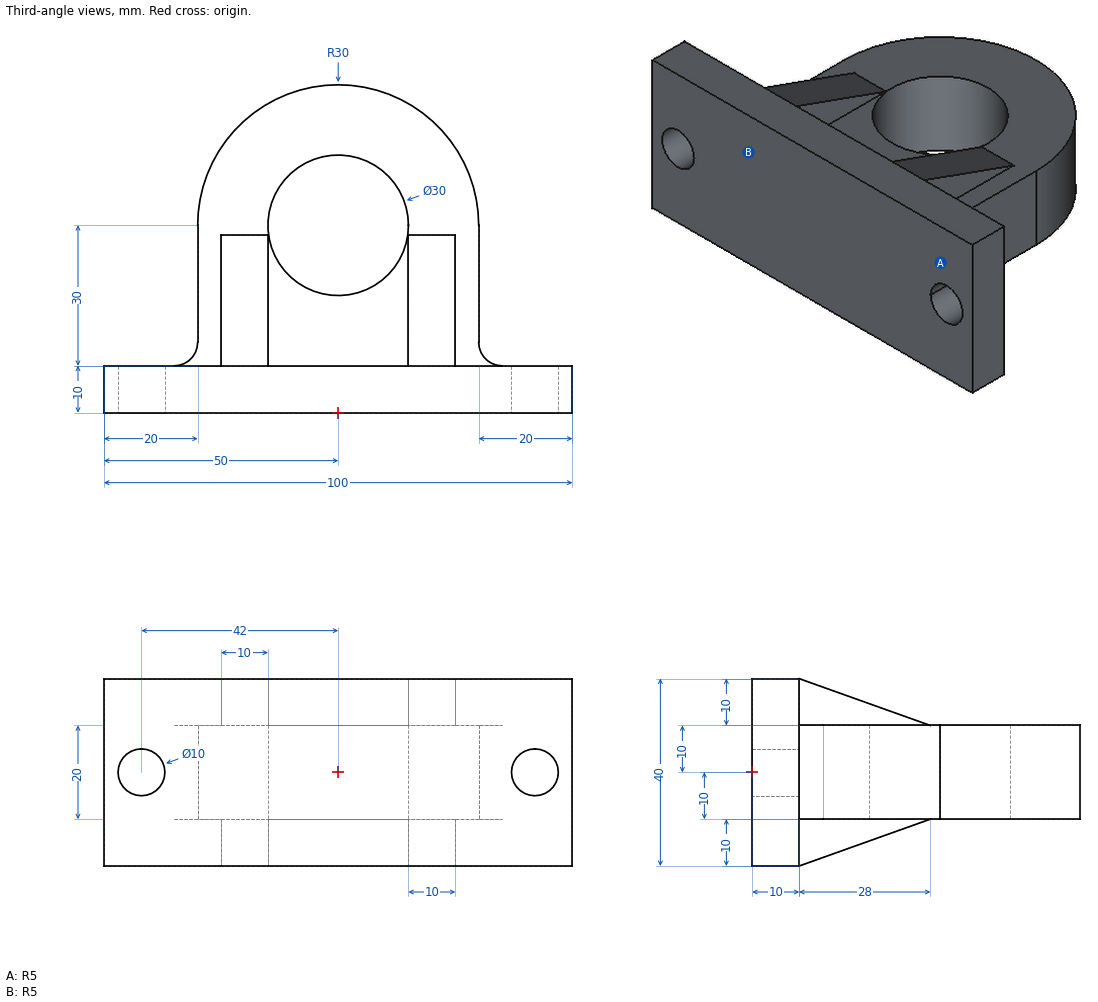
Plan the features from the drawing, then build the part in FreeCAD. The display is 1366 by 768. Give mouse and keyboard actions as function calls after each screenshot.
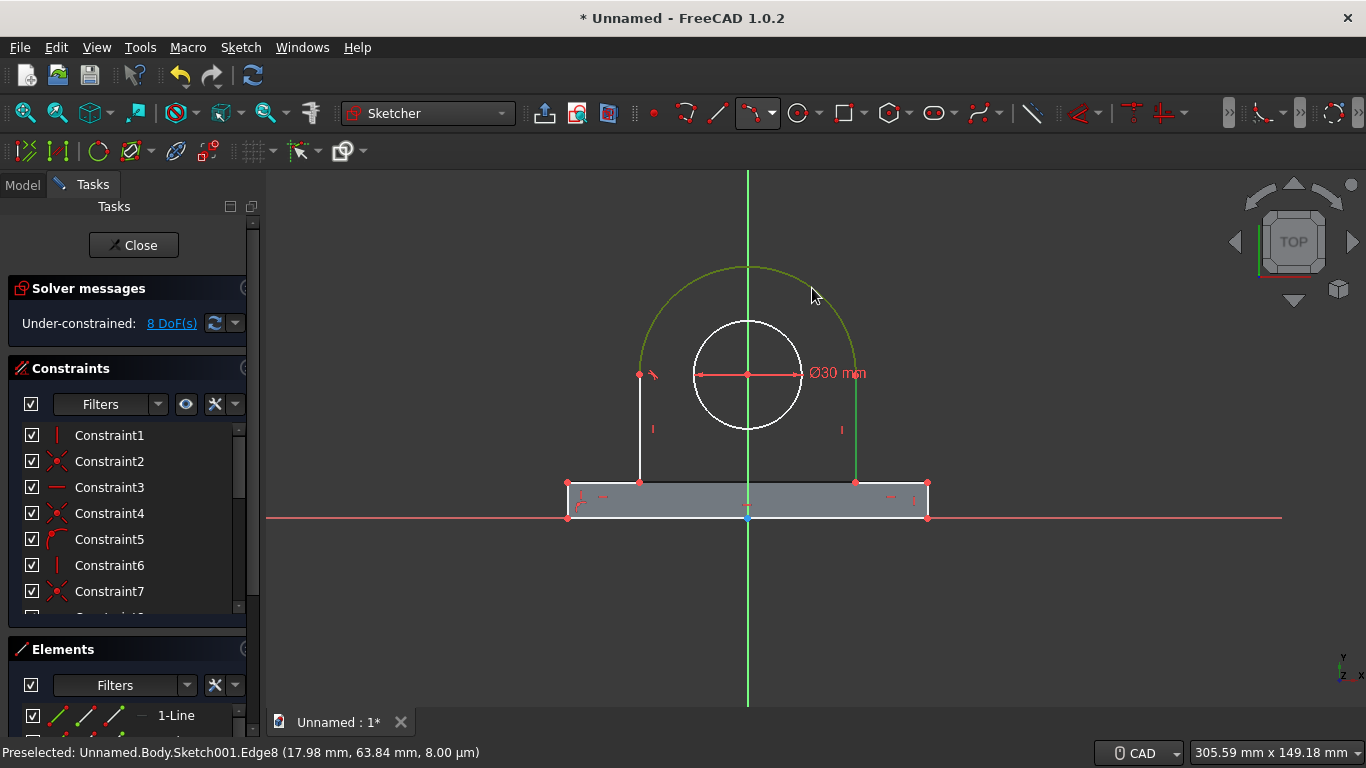
key(t)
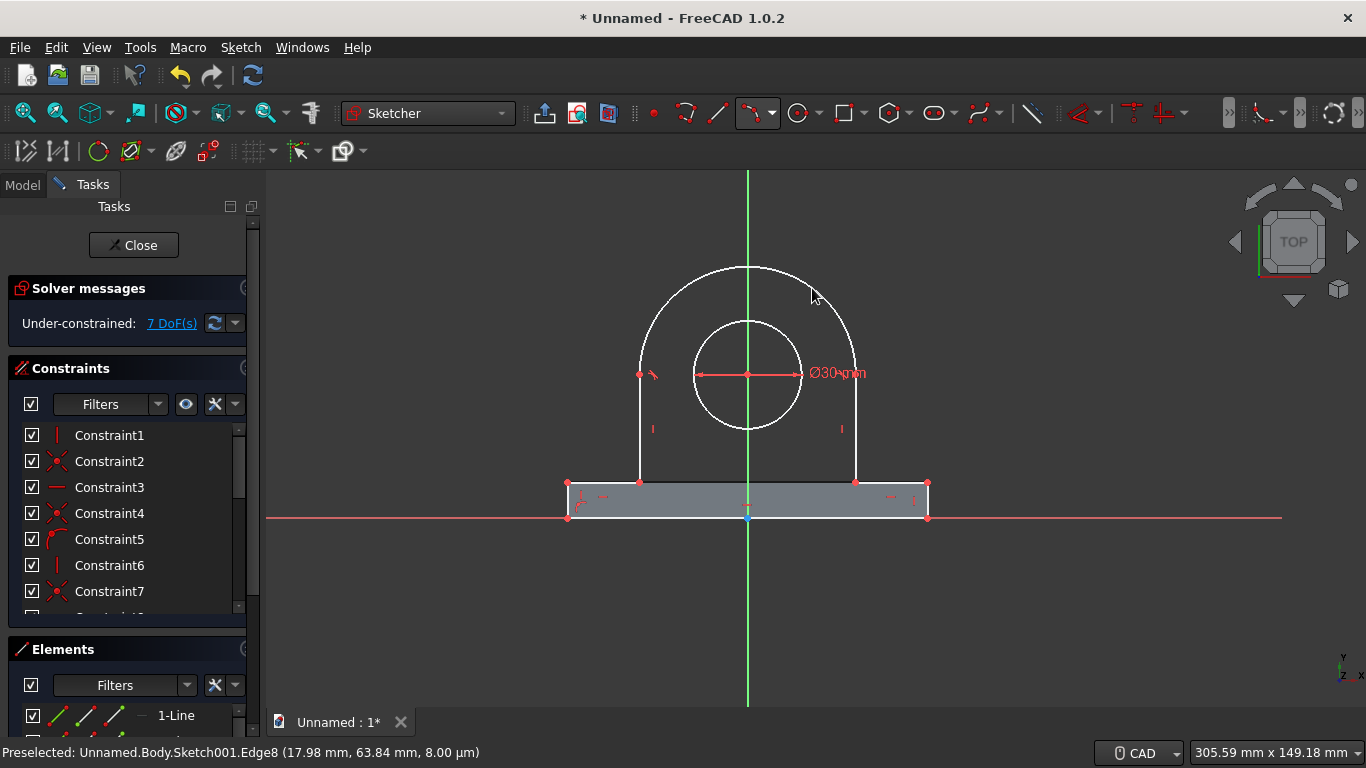
click(748, 375)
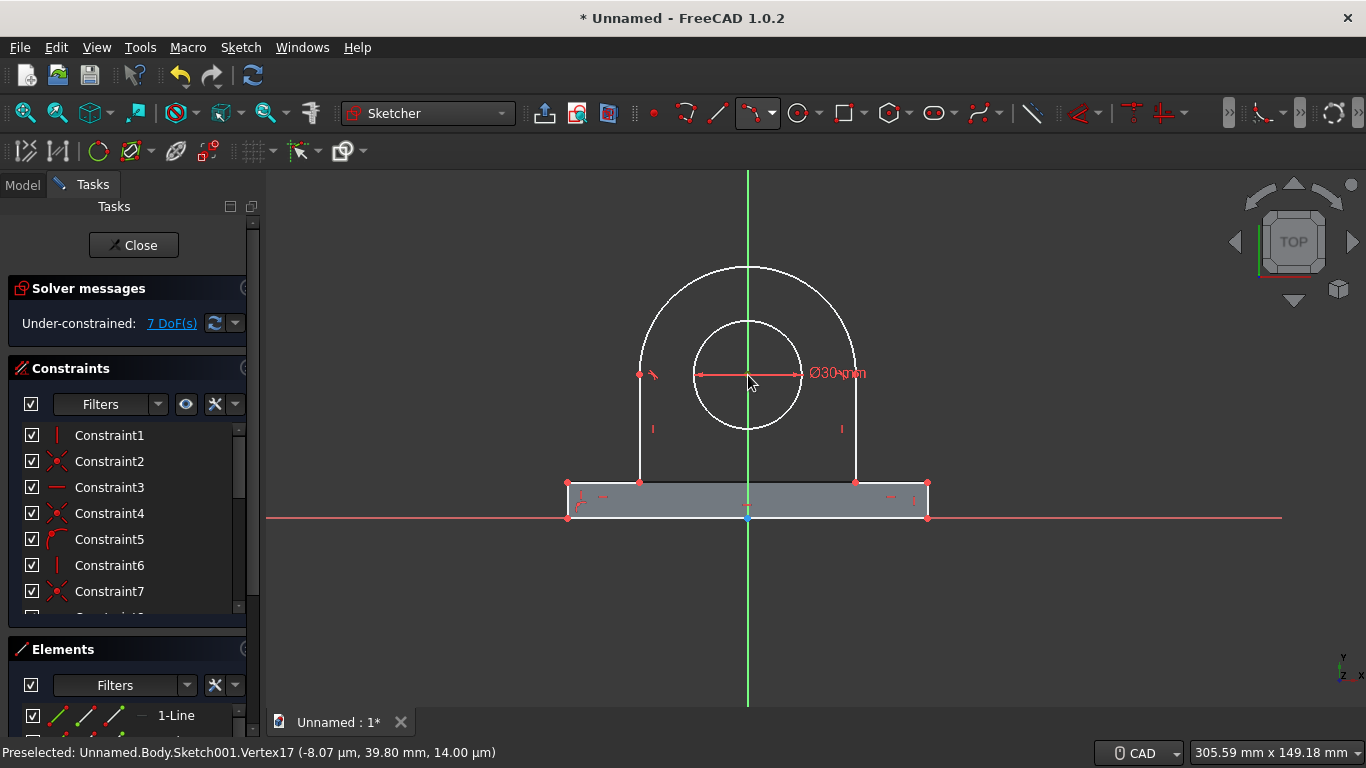
click(748, 645)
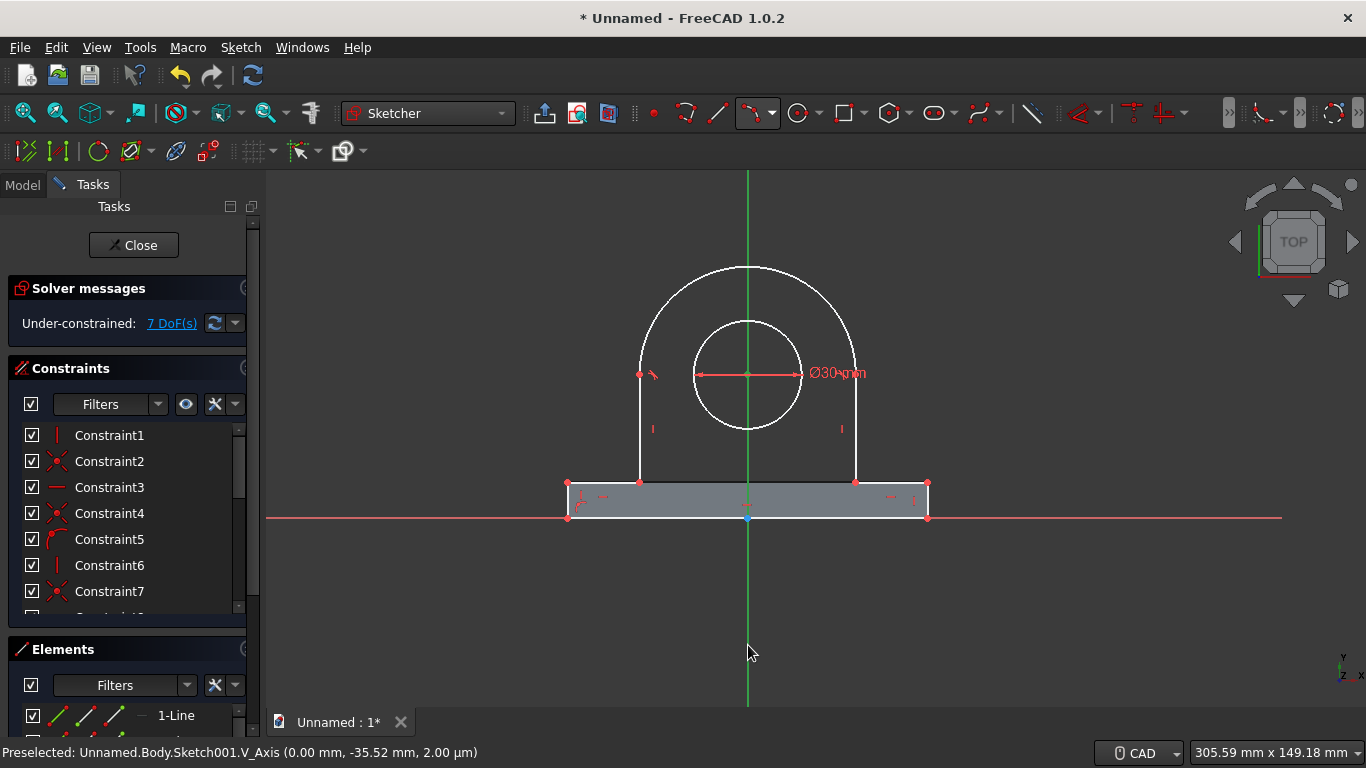
click(1132, 114)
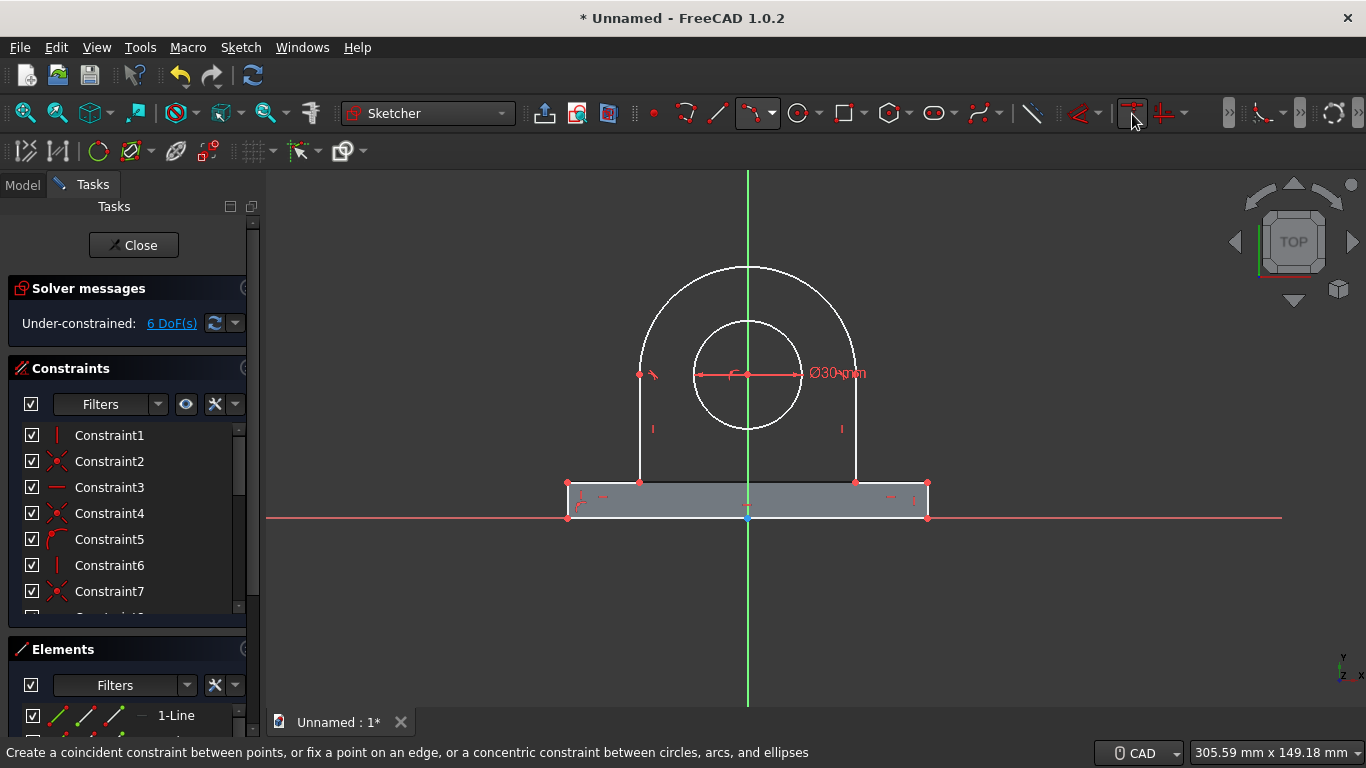
key(d)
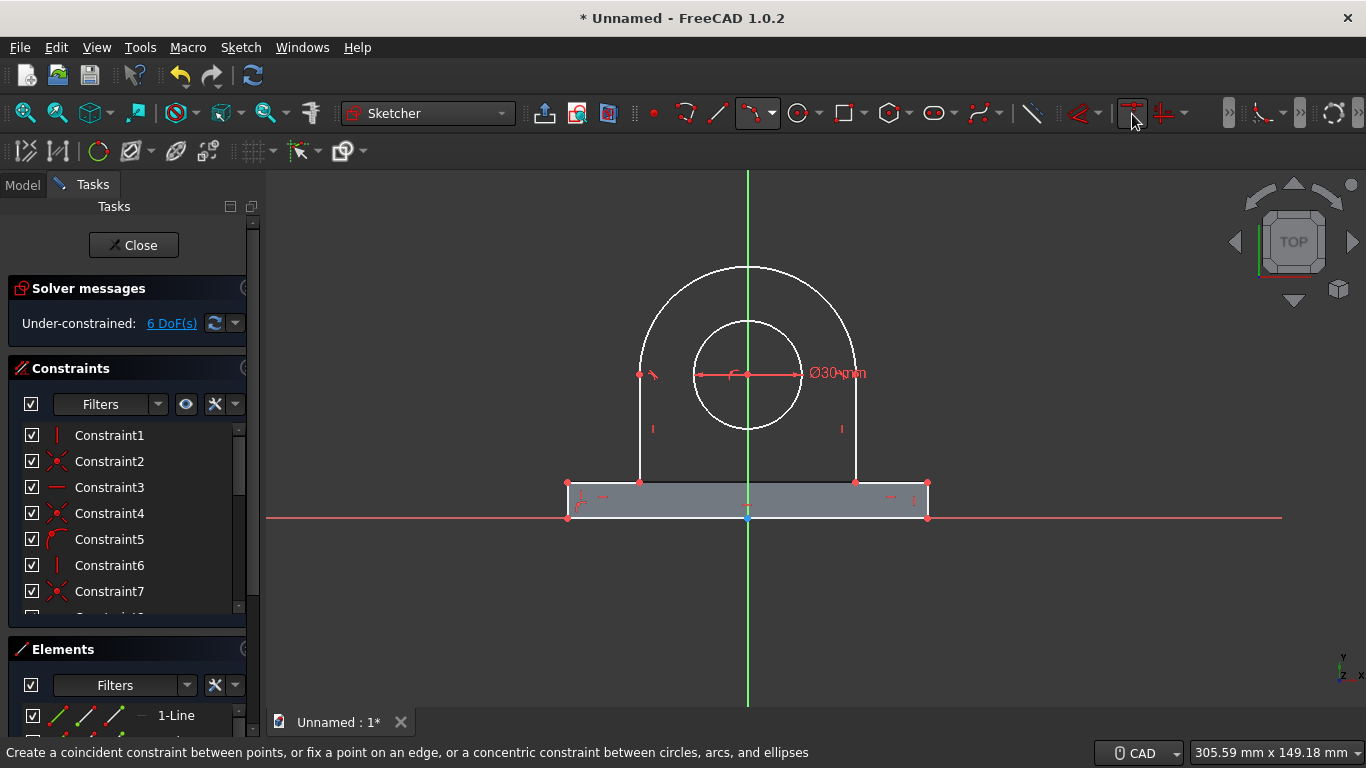
click(811, 287)
click(830, 261)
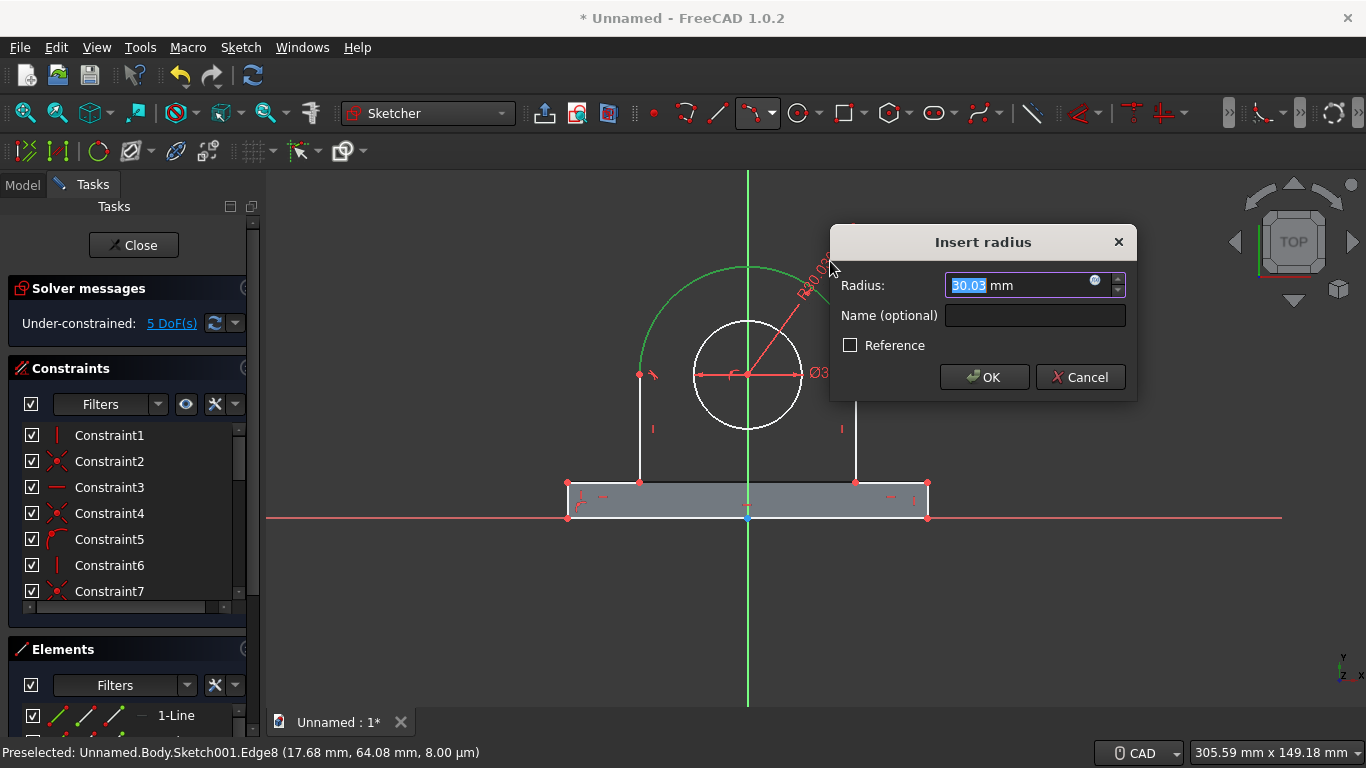
text(30)
key(Return)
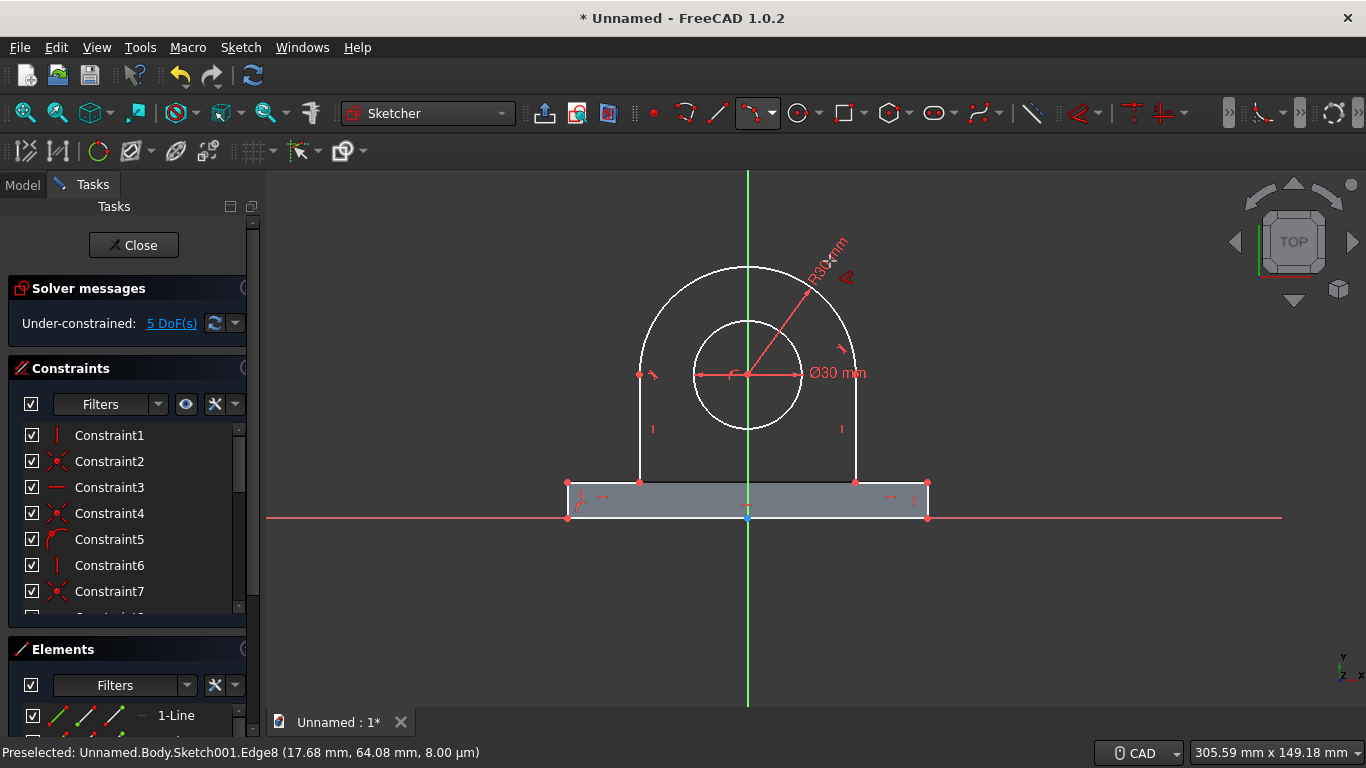
click(640, 407)
click(606, 429)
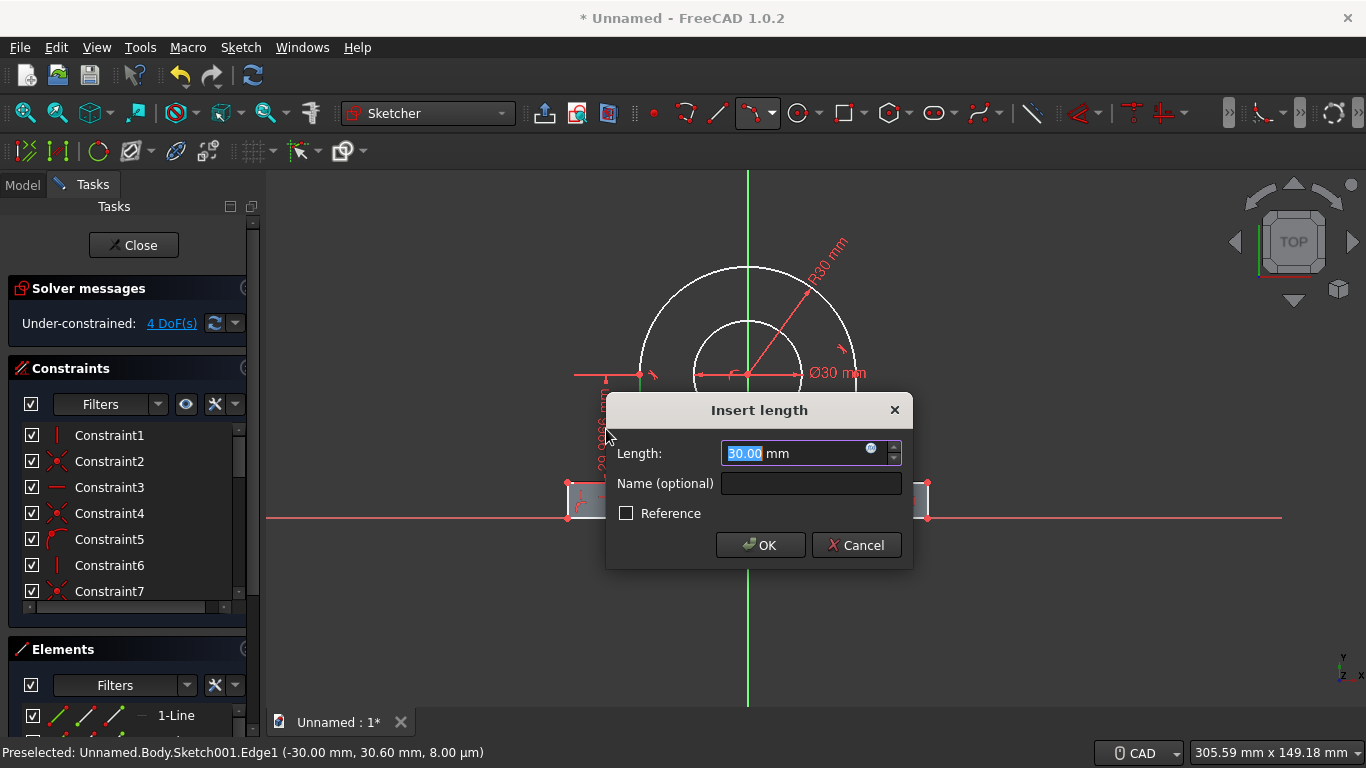
text(30)
key(Return)